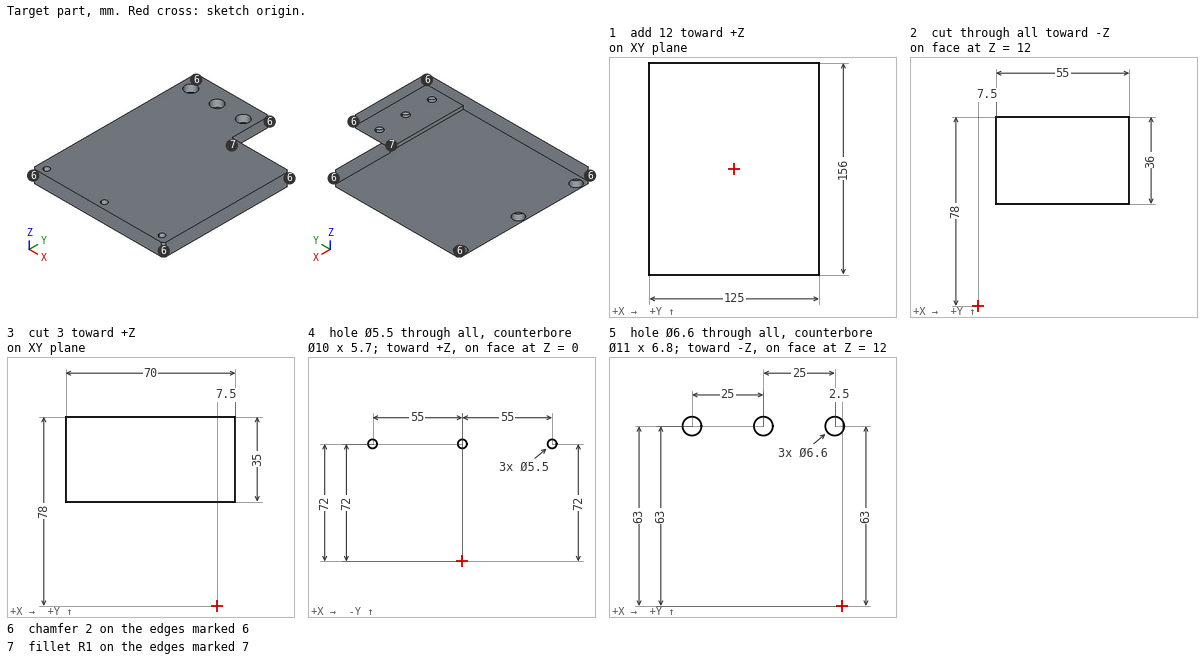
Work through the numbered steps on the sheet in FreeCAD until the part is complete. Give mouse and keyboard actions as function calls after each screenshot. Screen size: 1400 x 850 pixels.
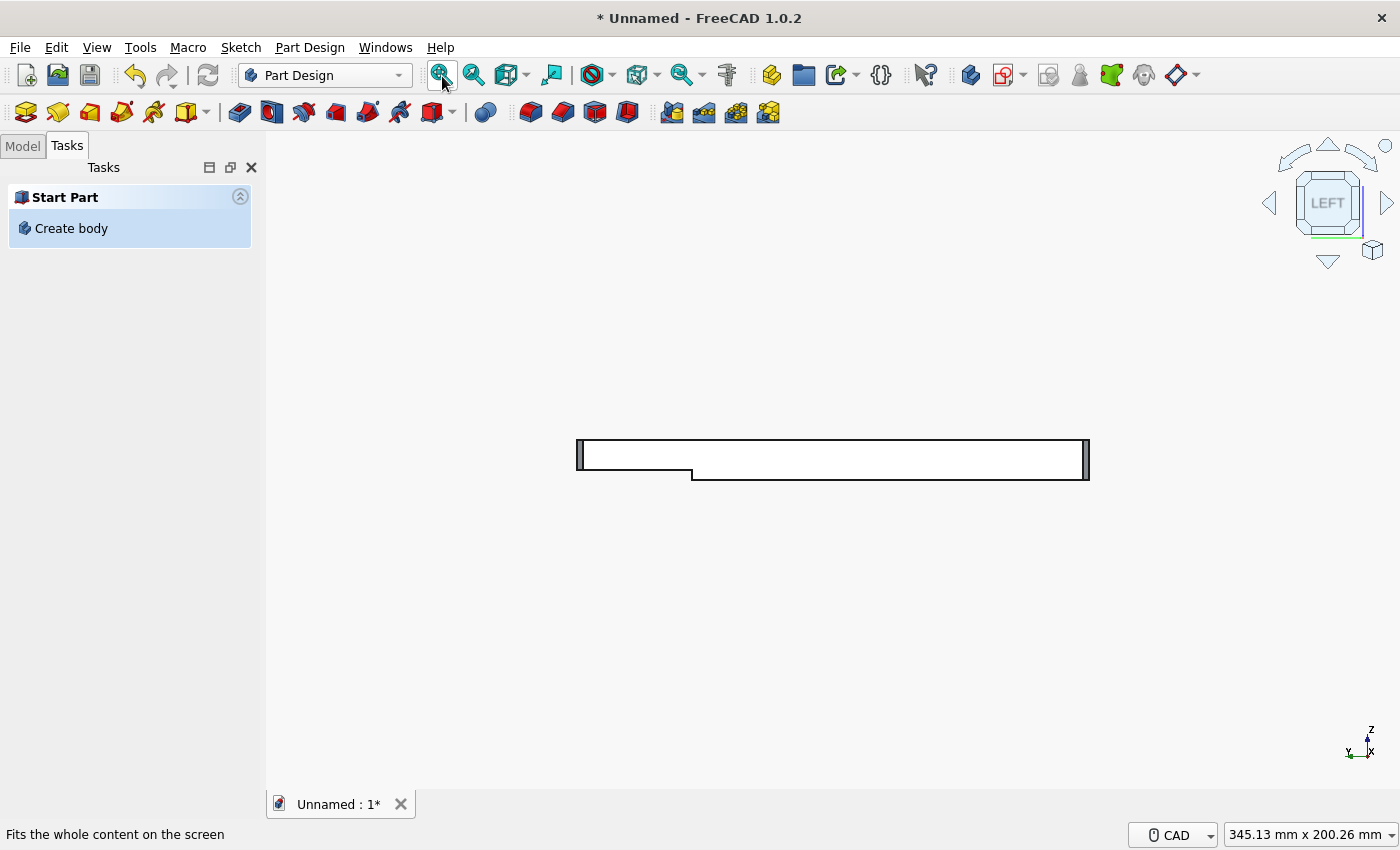
key(v)
key(3)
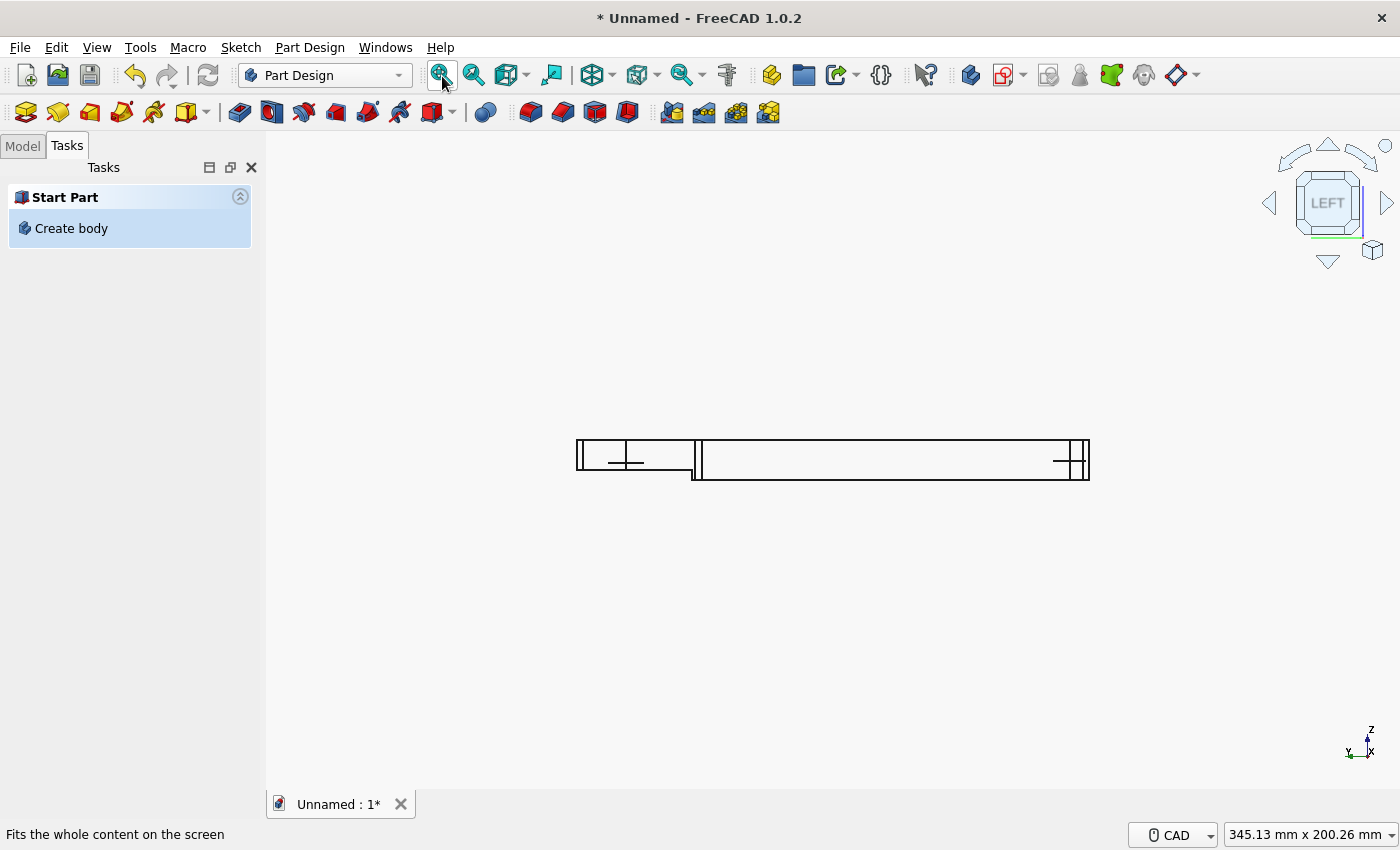
key(0)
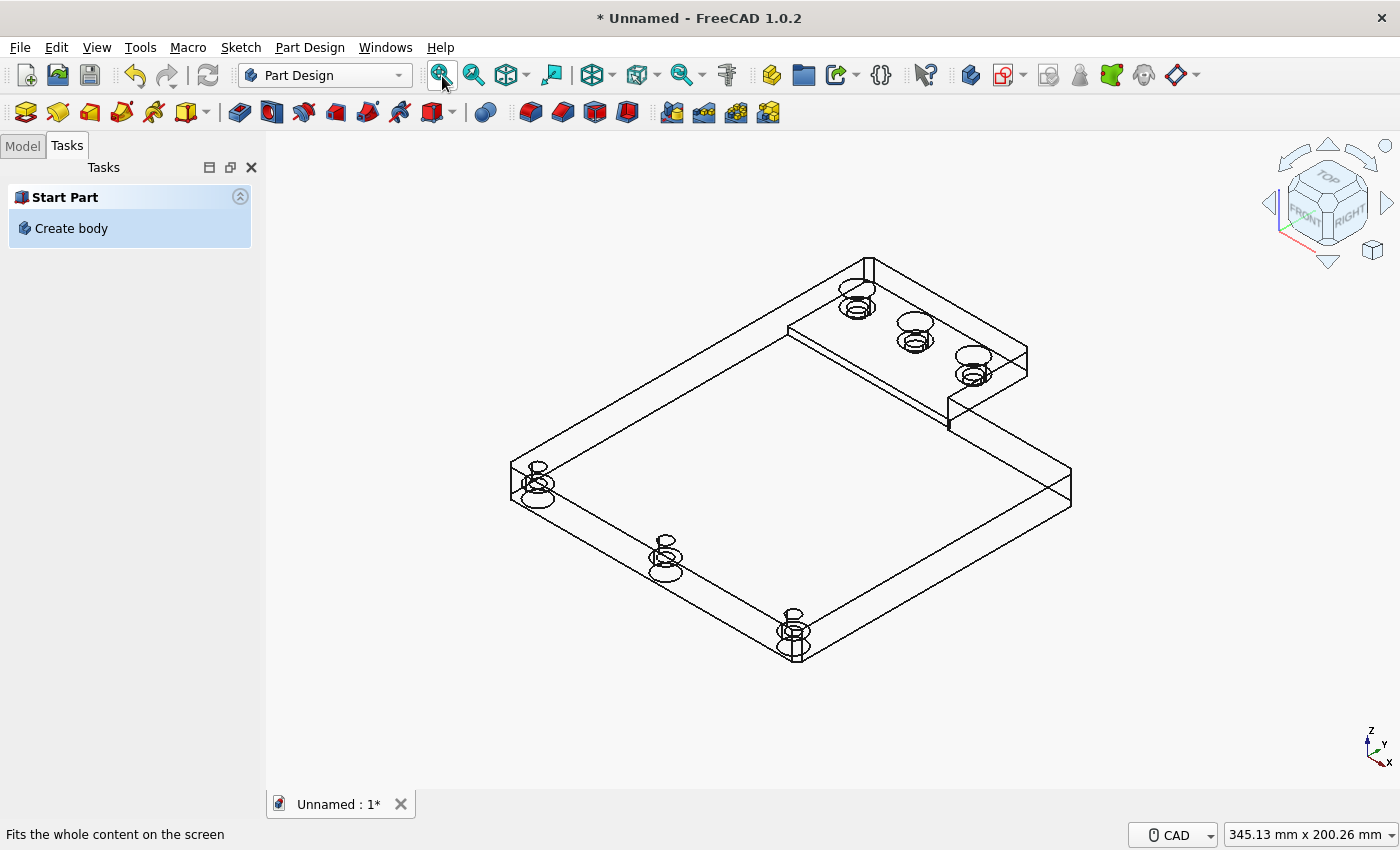
click(948, 413)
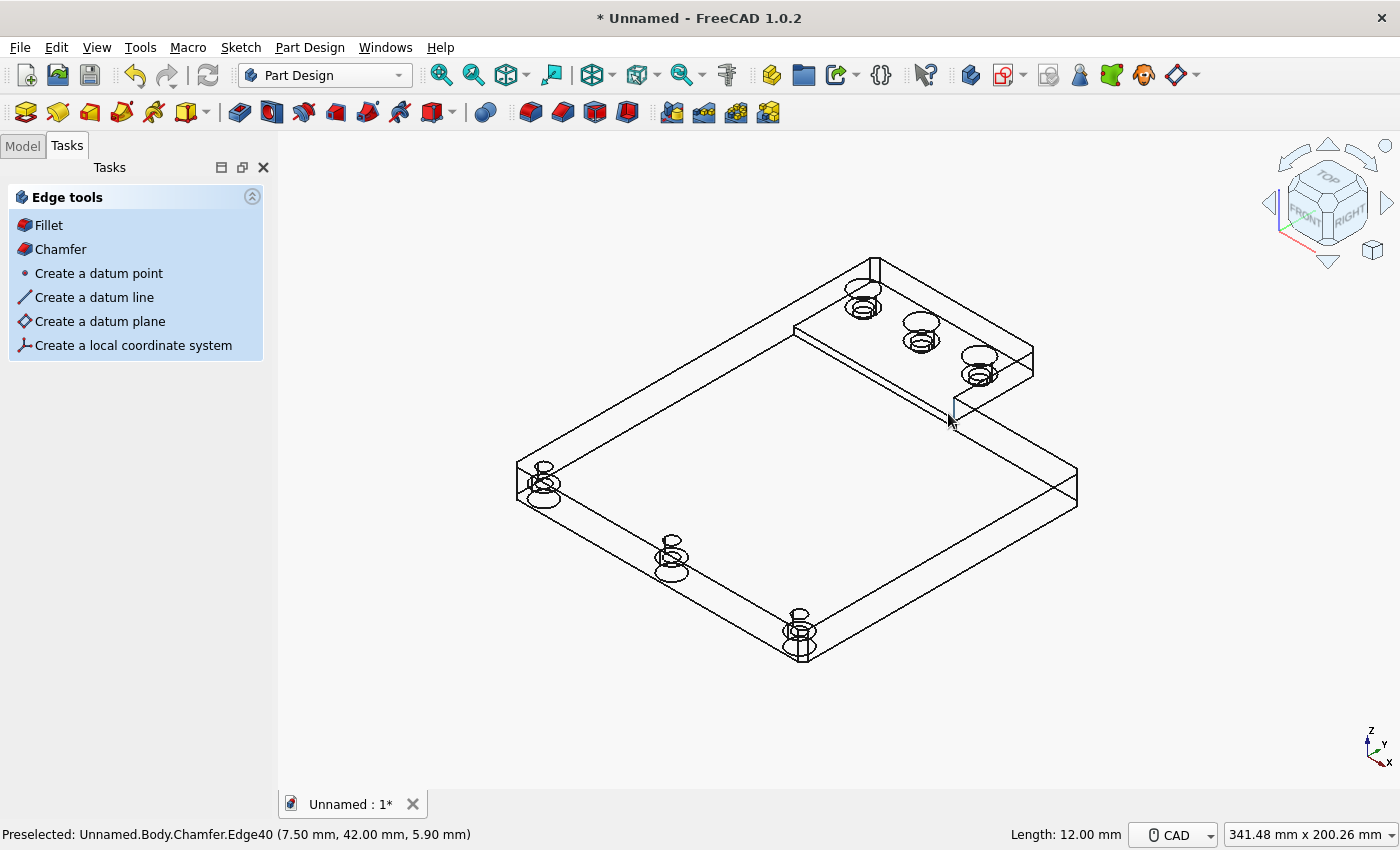
key(v)
key(1)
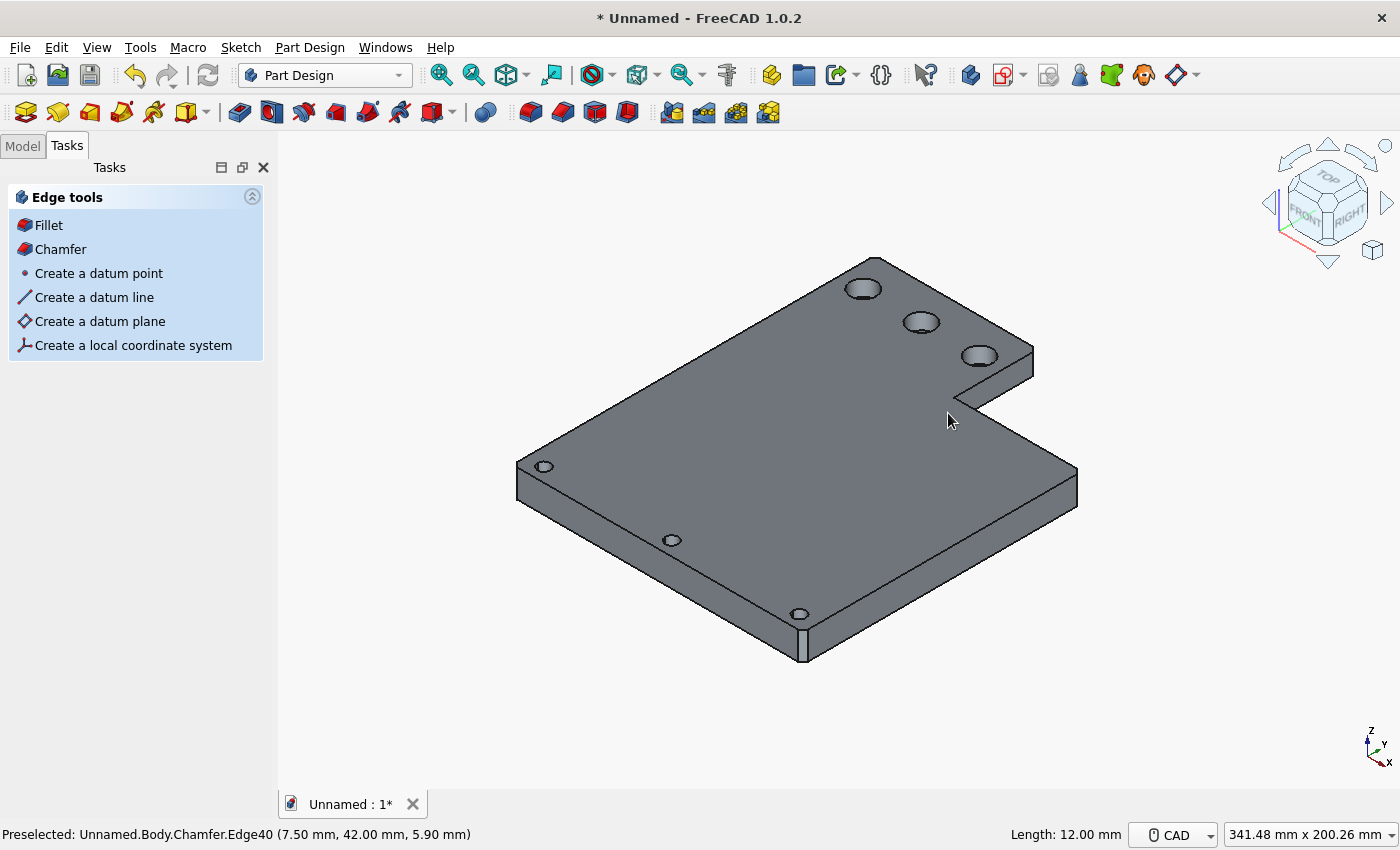
click(532, 112)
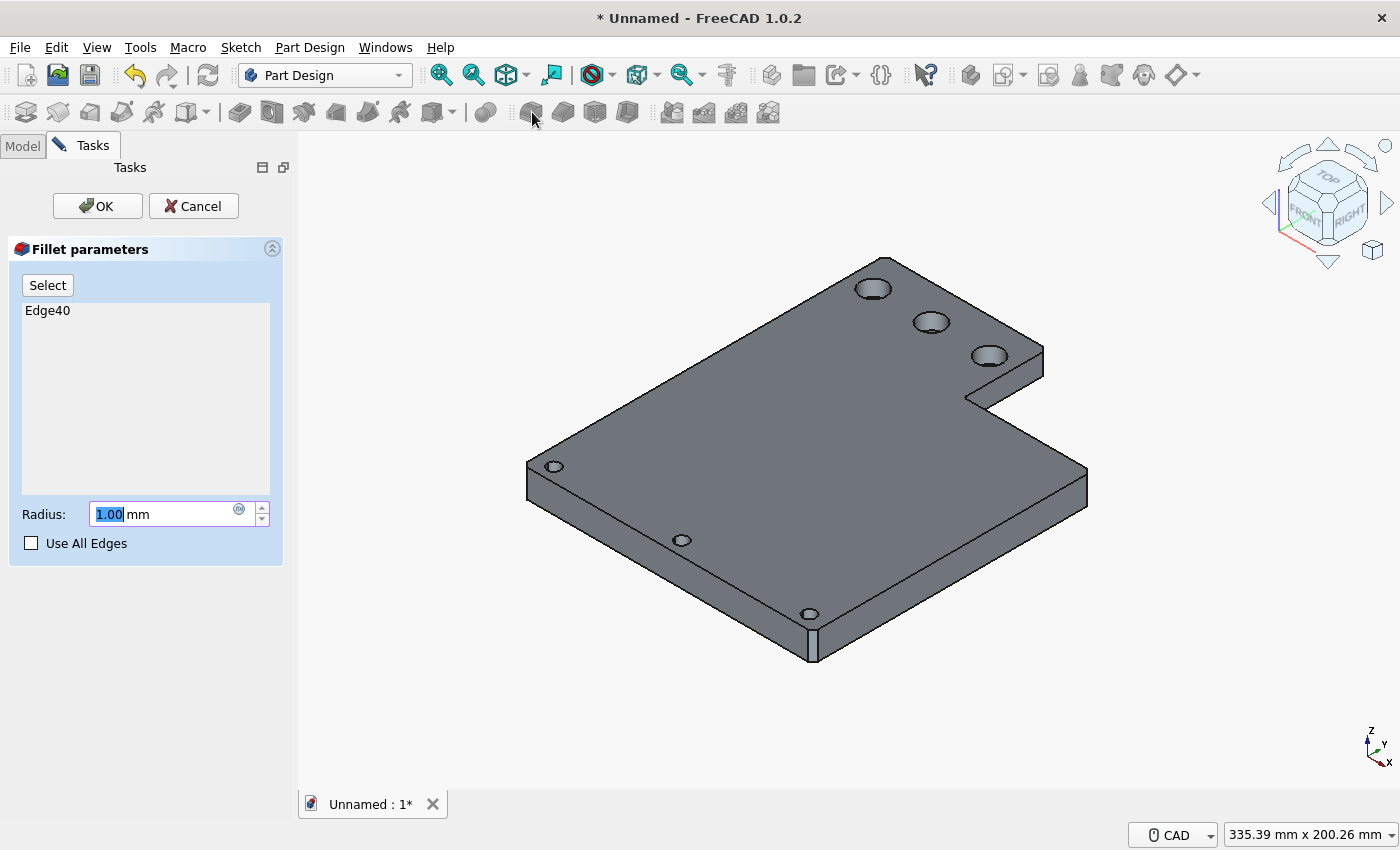
text(1)
key(Tab)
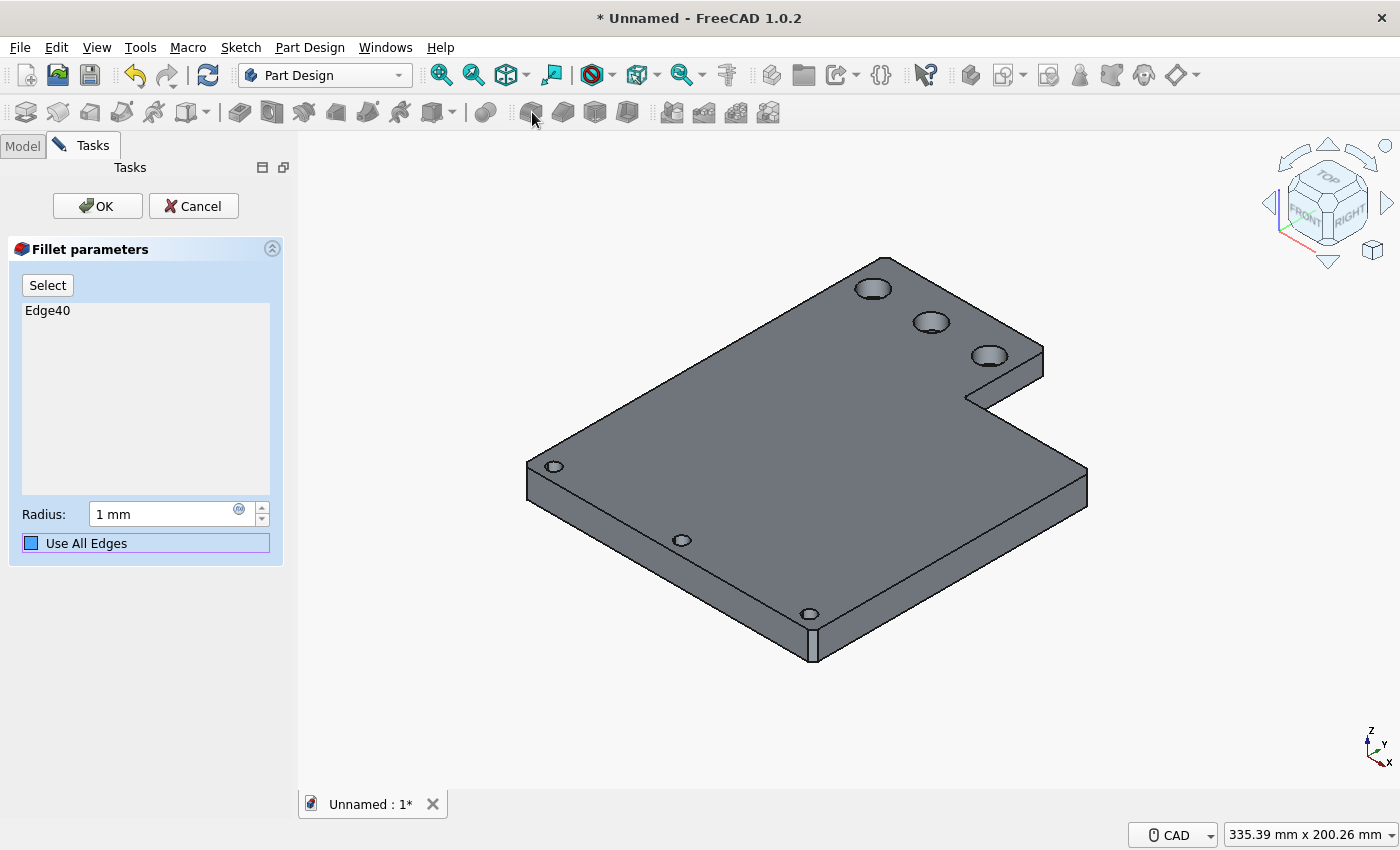
click(98, 206)